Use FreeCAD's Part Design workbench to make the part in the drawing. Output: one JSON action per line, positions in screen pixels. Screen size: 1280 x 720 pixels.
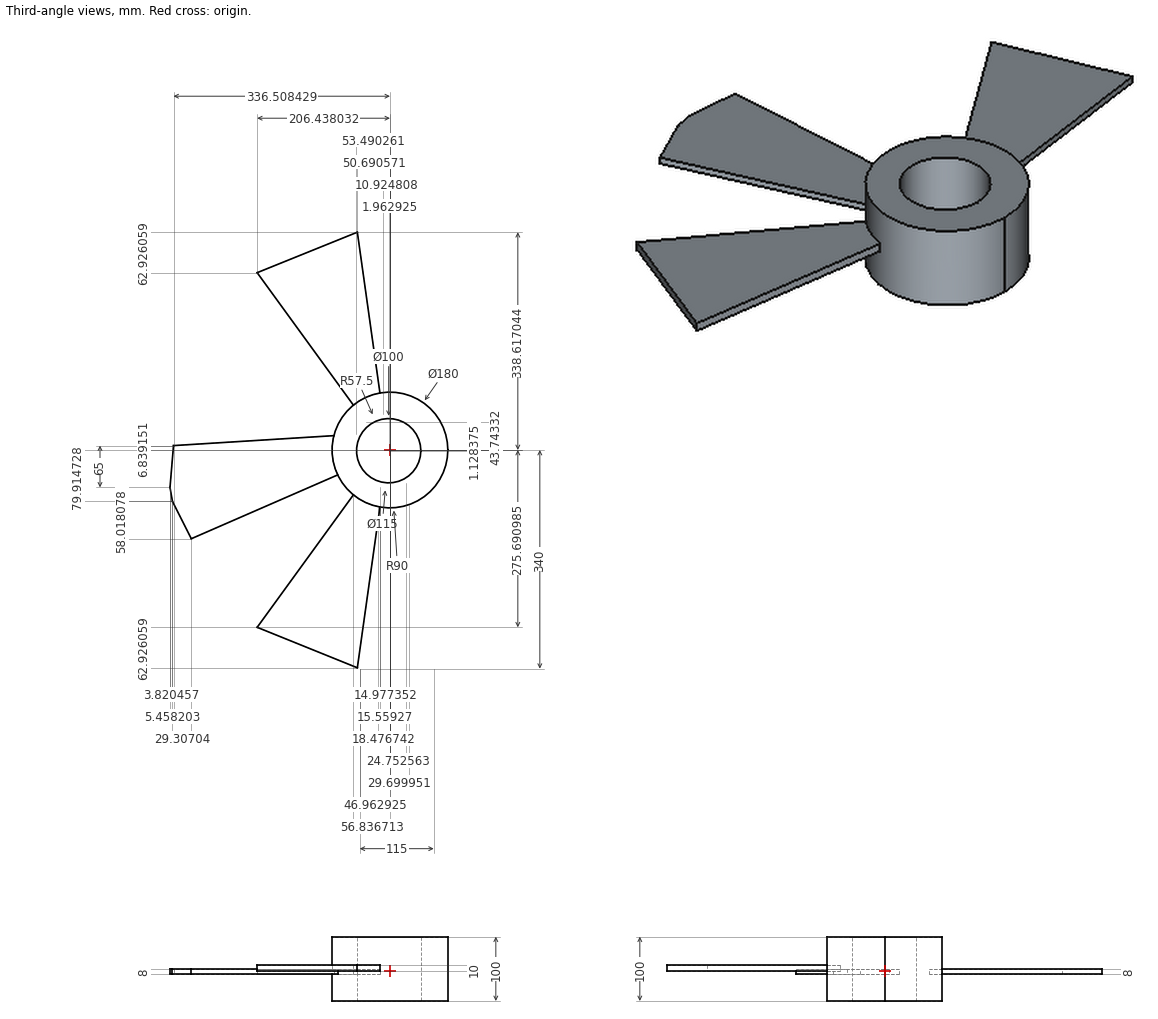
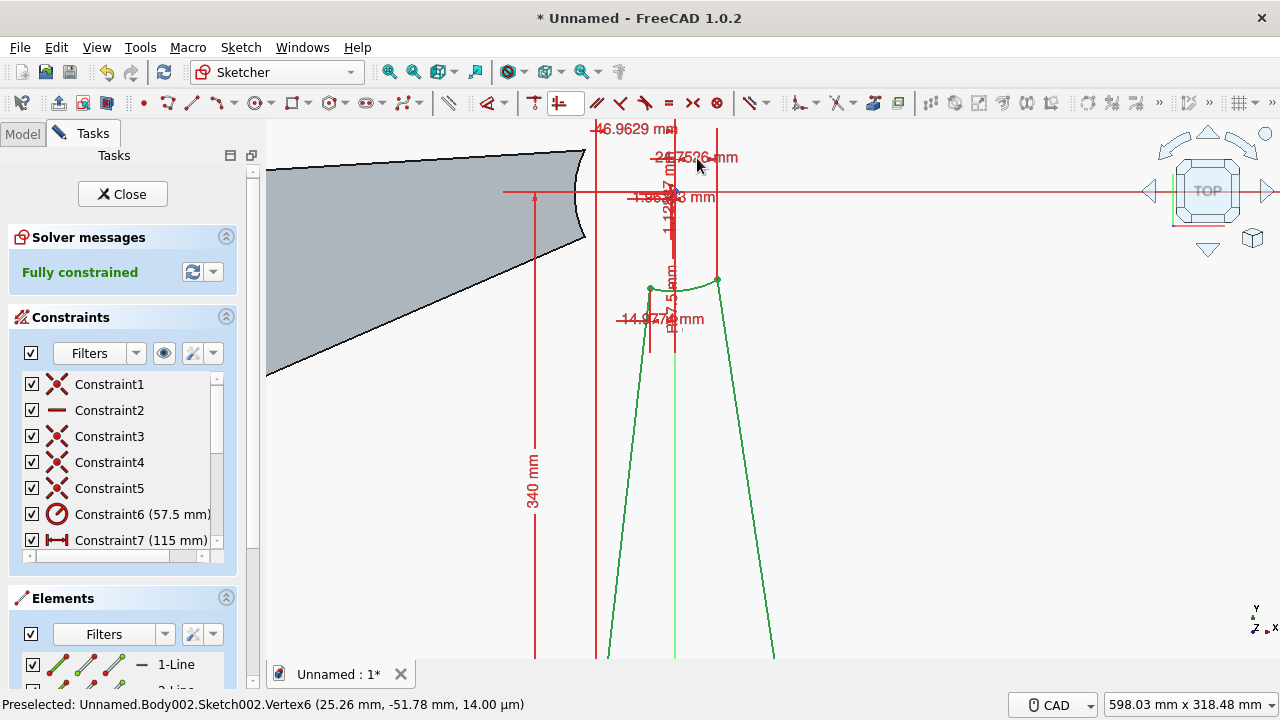
{"action": "left_click", "coordinate": [123, 194]}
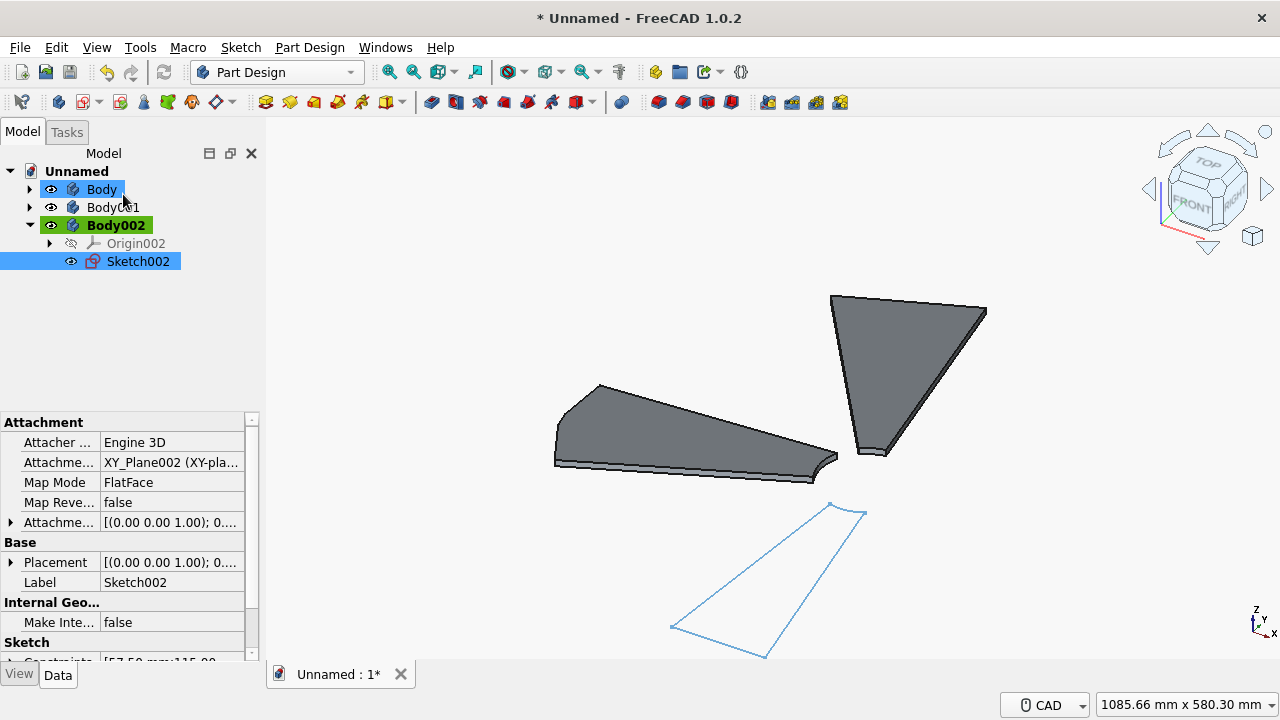
{"action": "left_click", "coordinate": [266, 102]}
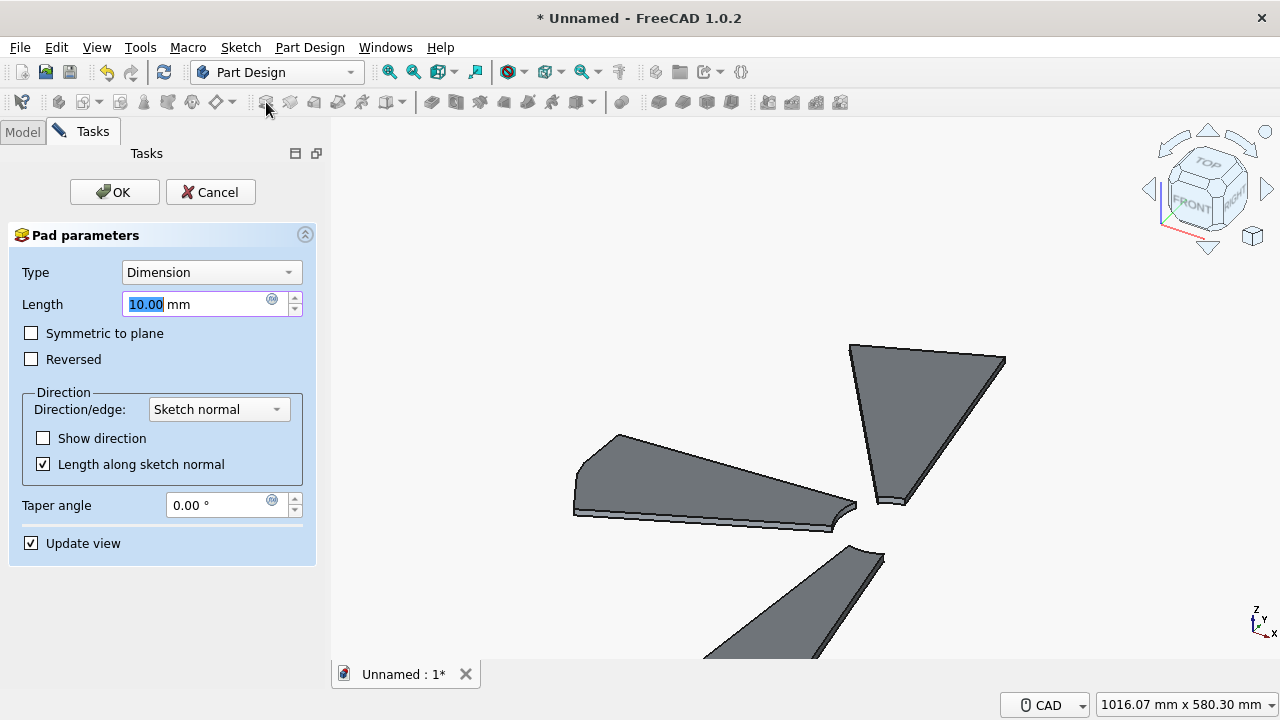
{"action": "type", "text": "8"}
{"action": "key", "text": "Tab"}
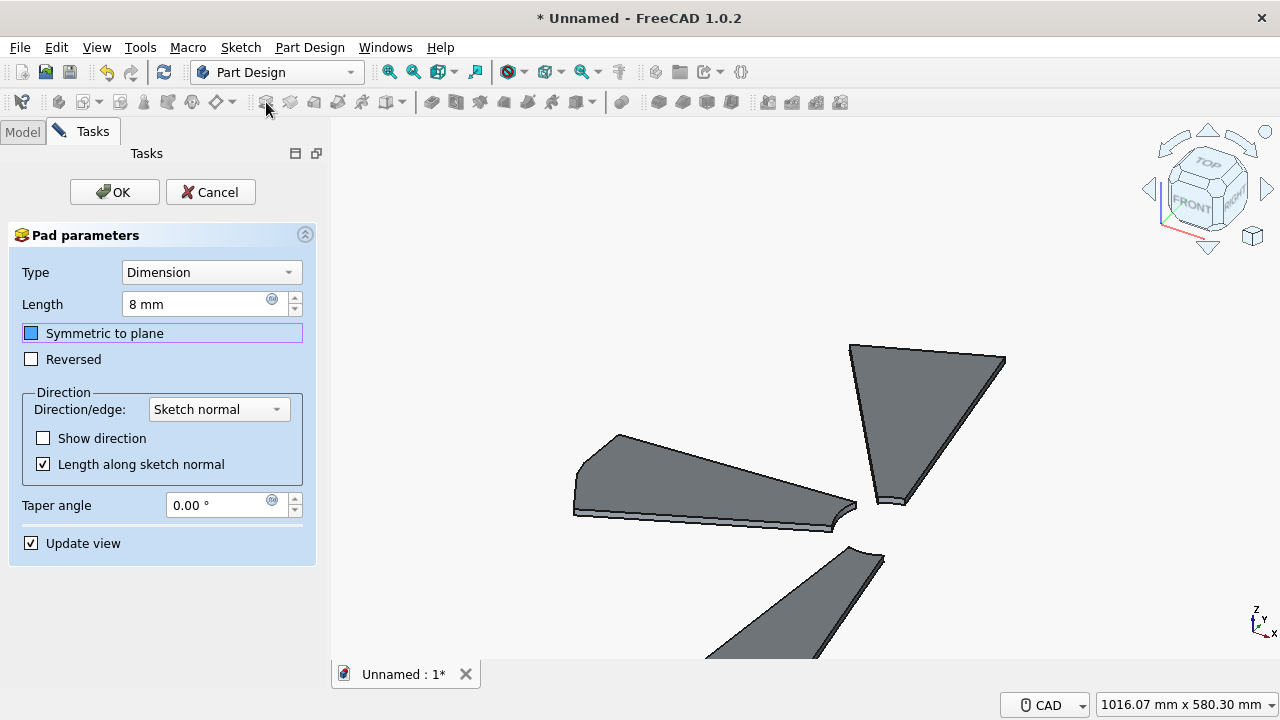
{"action": "left_click", "coordinate": [30, 333]}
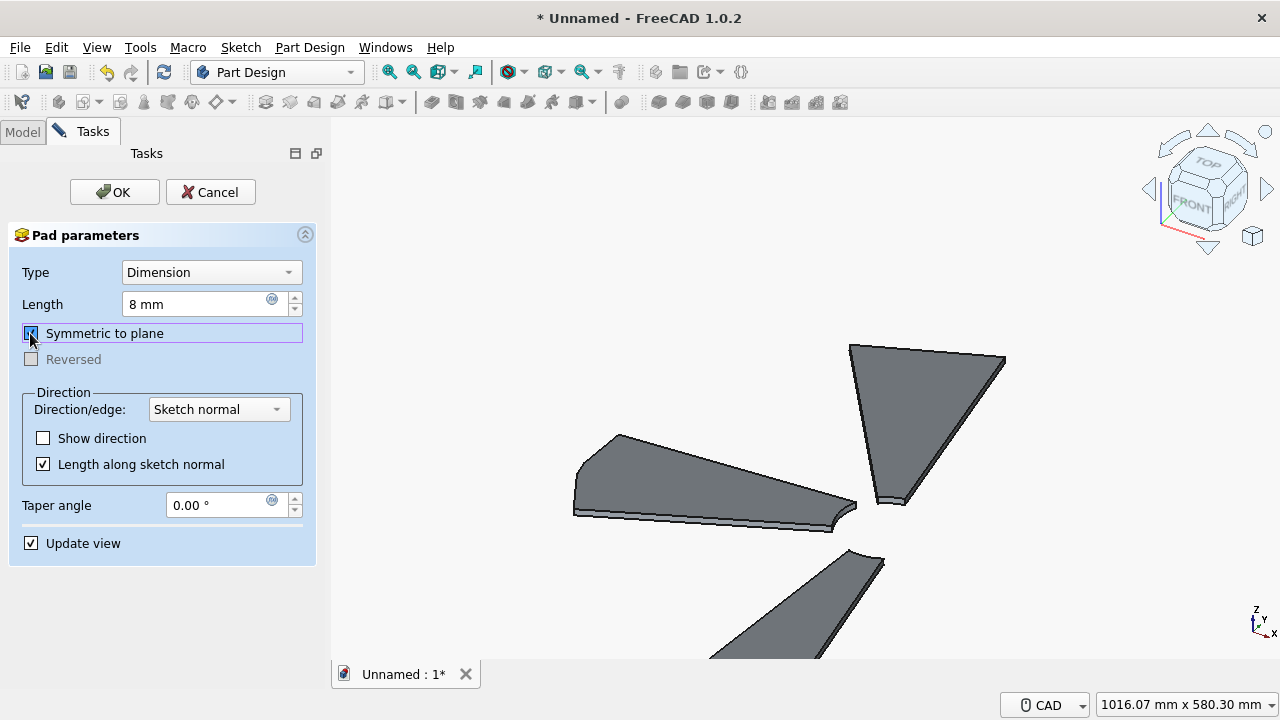
{"action": "left_click", "coordinate": [115, 192]}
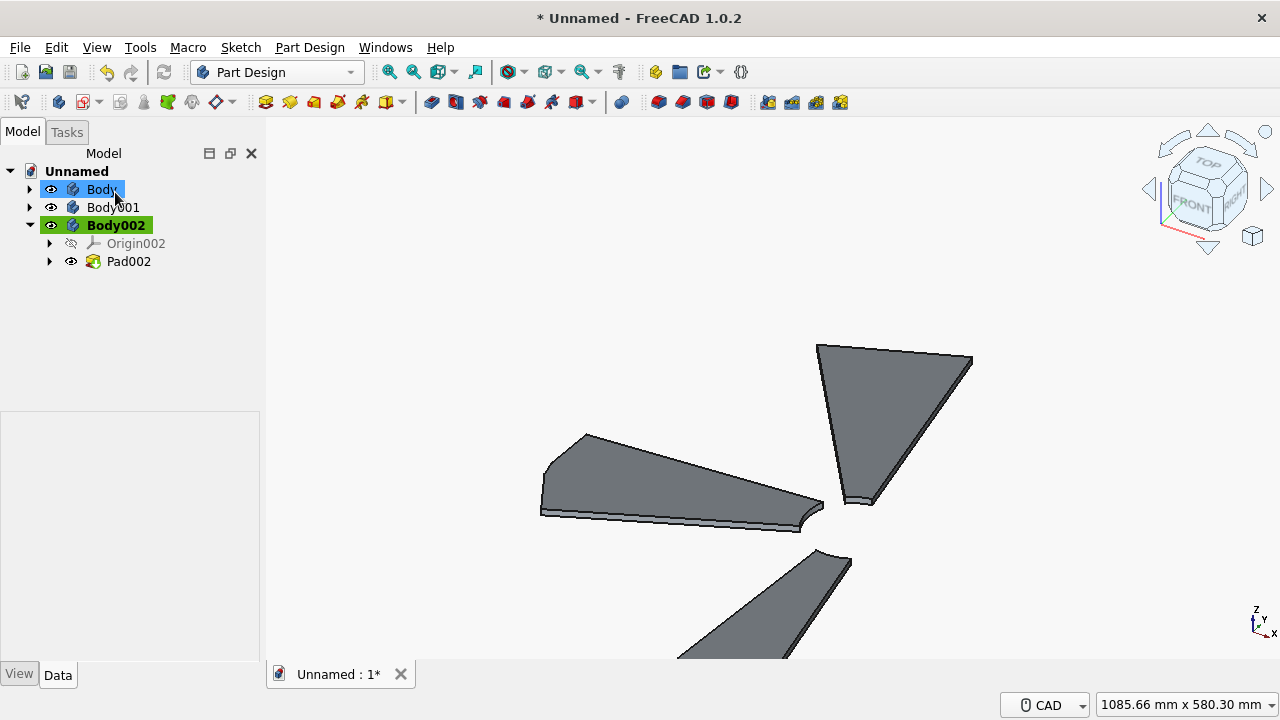
{"action": "left_click", "coordinate": [390, 72]}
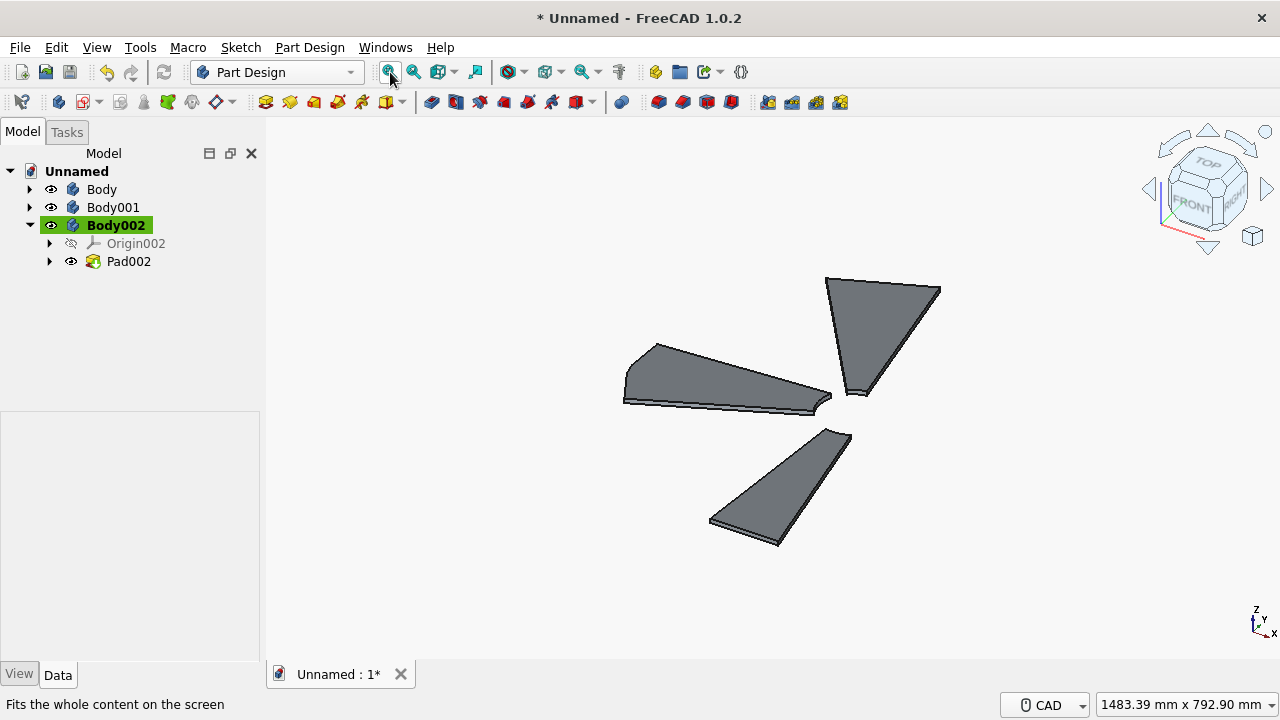
{"action": "double_click", "coordinate": [96, 189]}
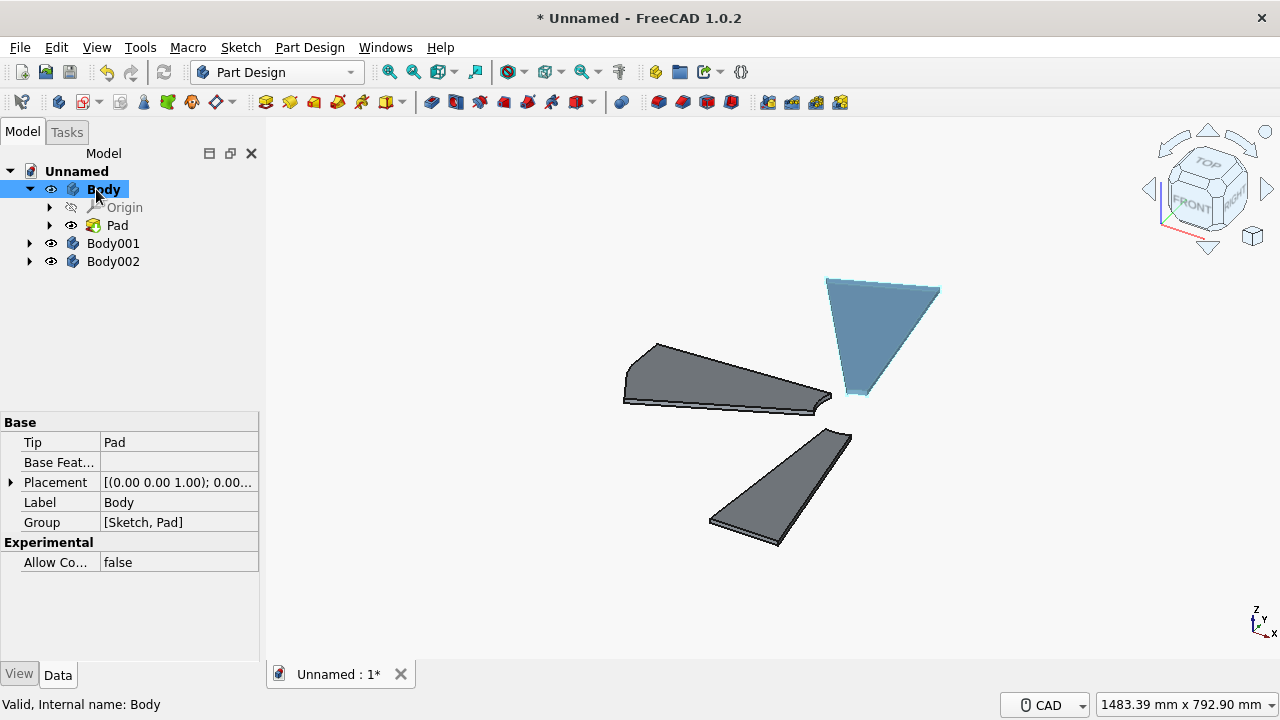
{"action": "left_click", "coordinate": [96, 189]}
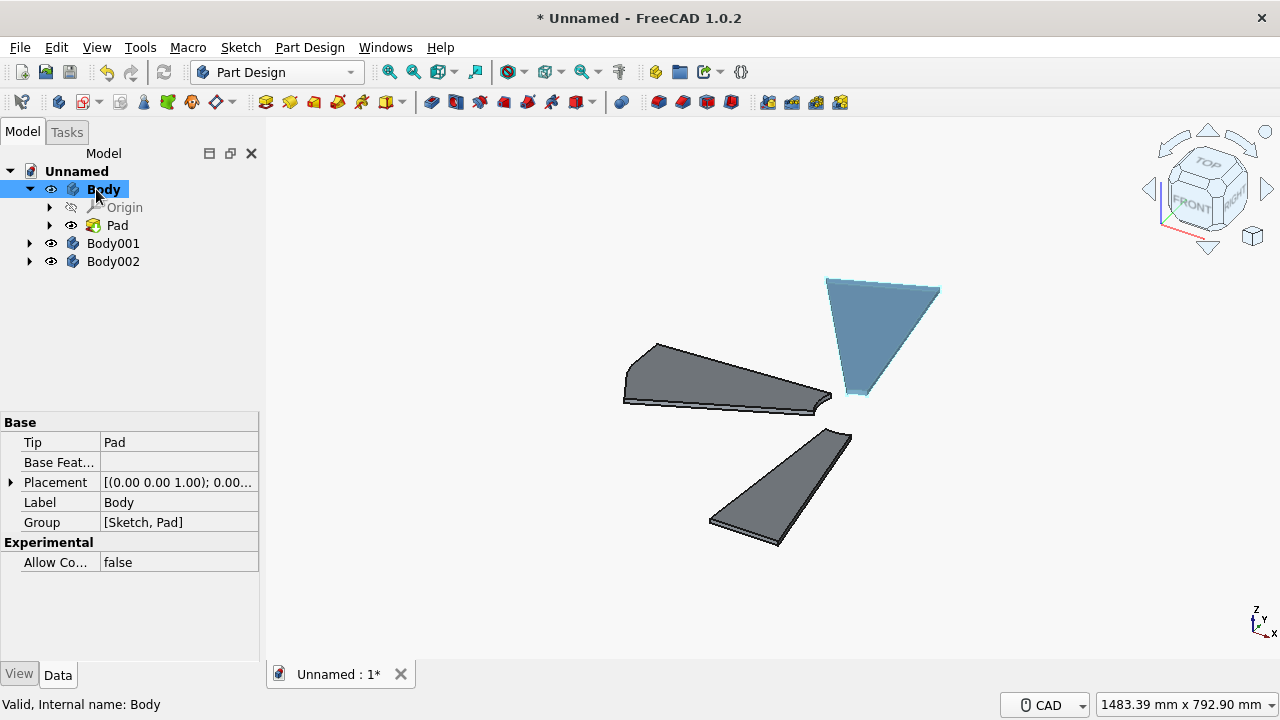
{"action": "left_click", "coordinate": [146, 562]}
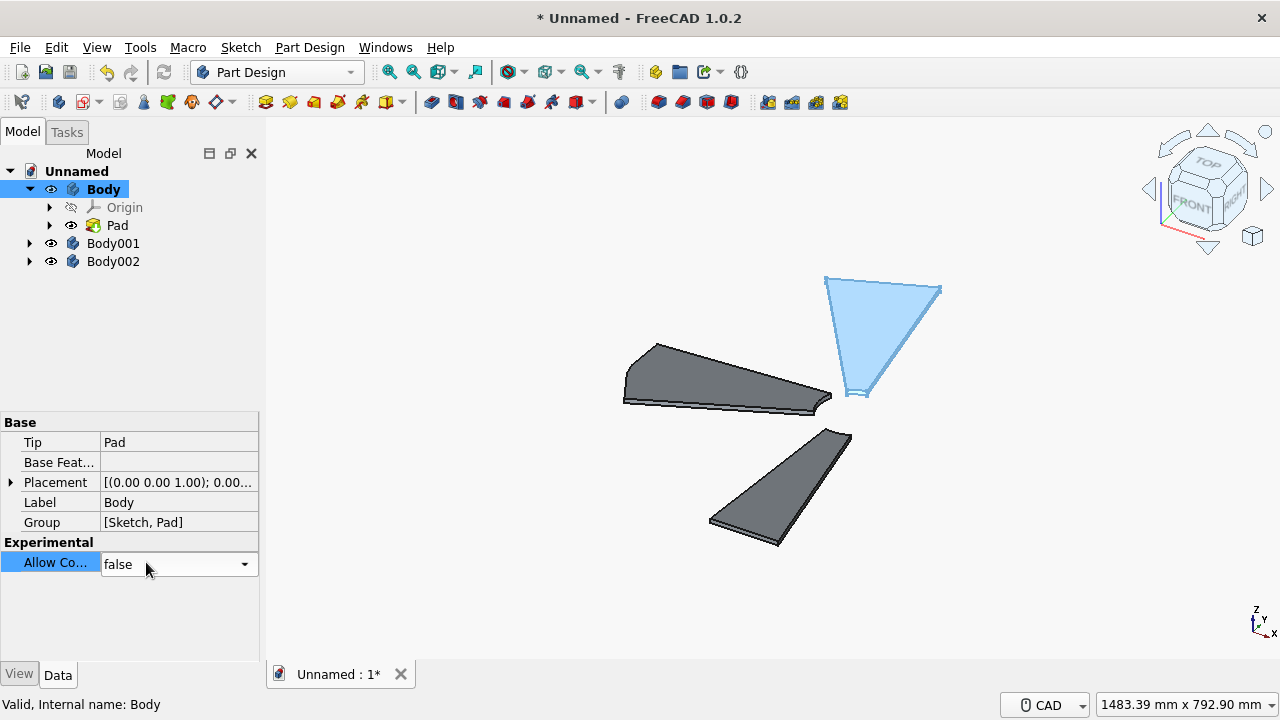
{"action": "left_click", "coordinate": [146, 562]}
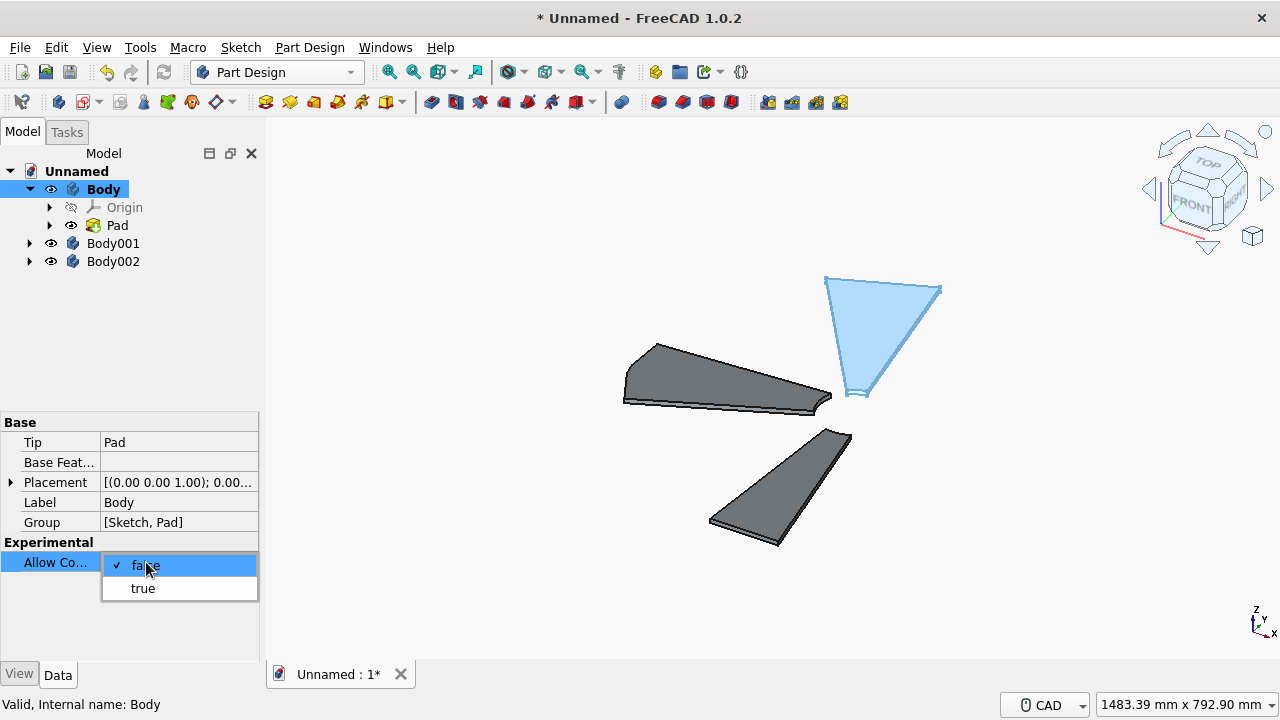
{"action": "left_click", "coordinate": [179, 588]}
{"action": "key", "text": "Return"}